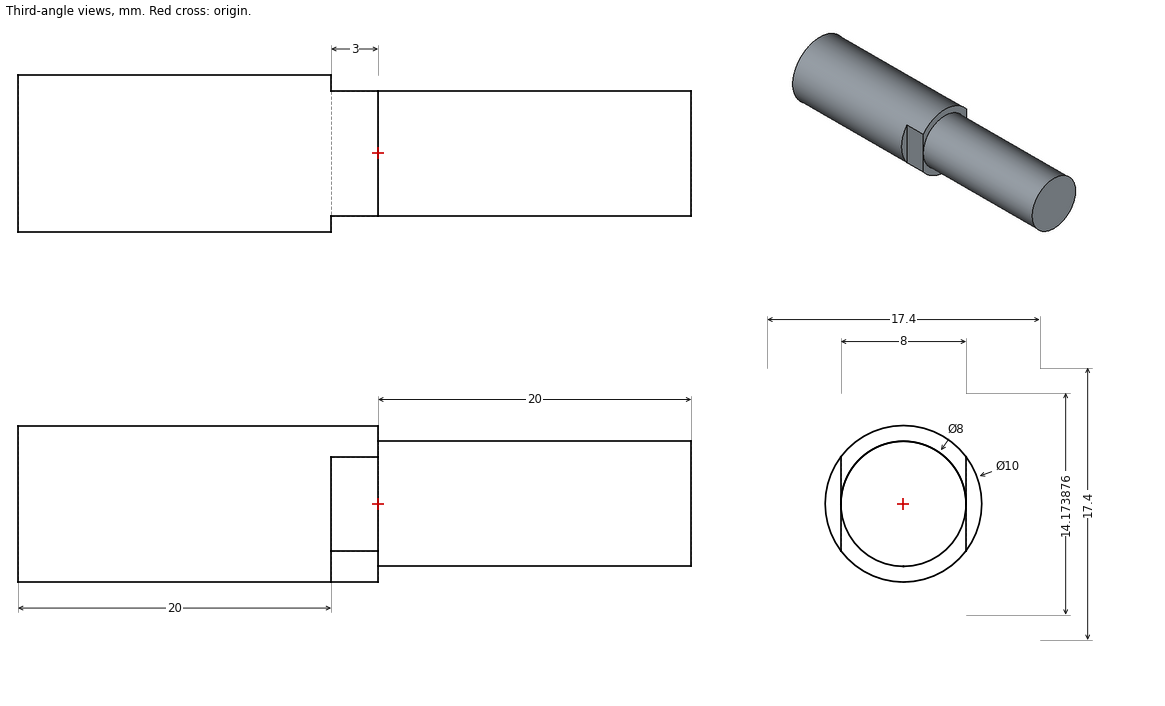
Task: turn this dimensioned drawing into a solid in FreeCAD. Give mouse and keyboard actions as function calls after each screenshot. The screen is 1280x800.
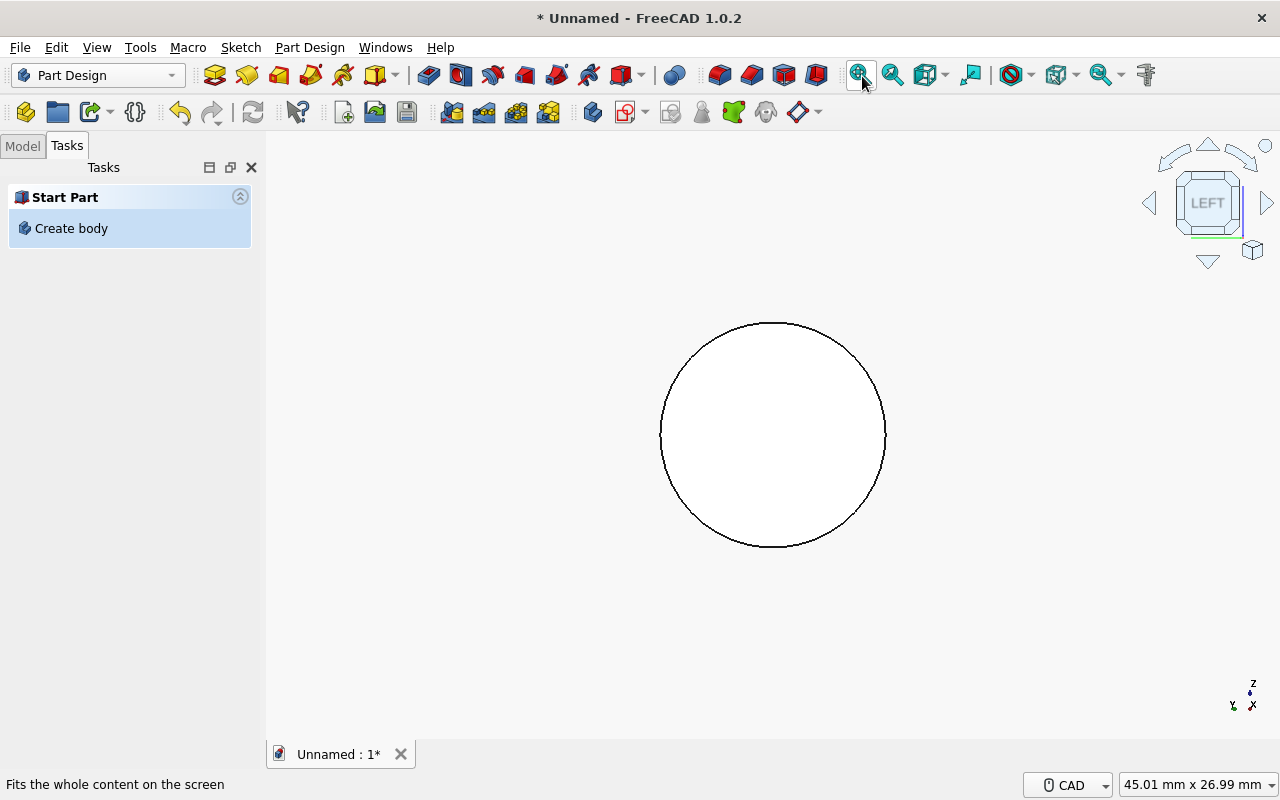
click(773, 434)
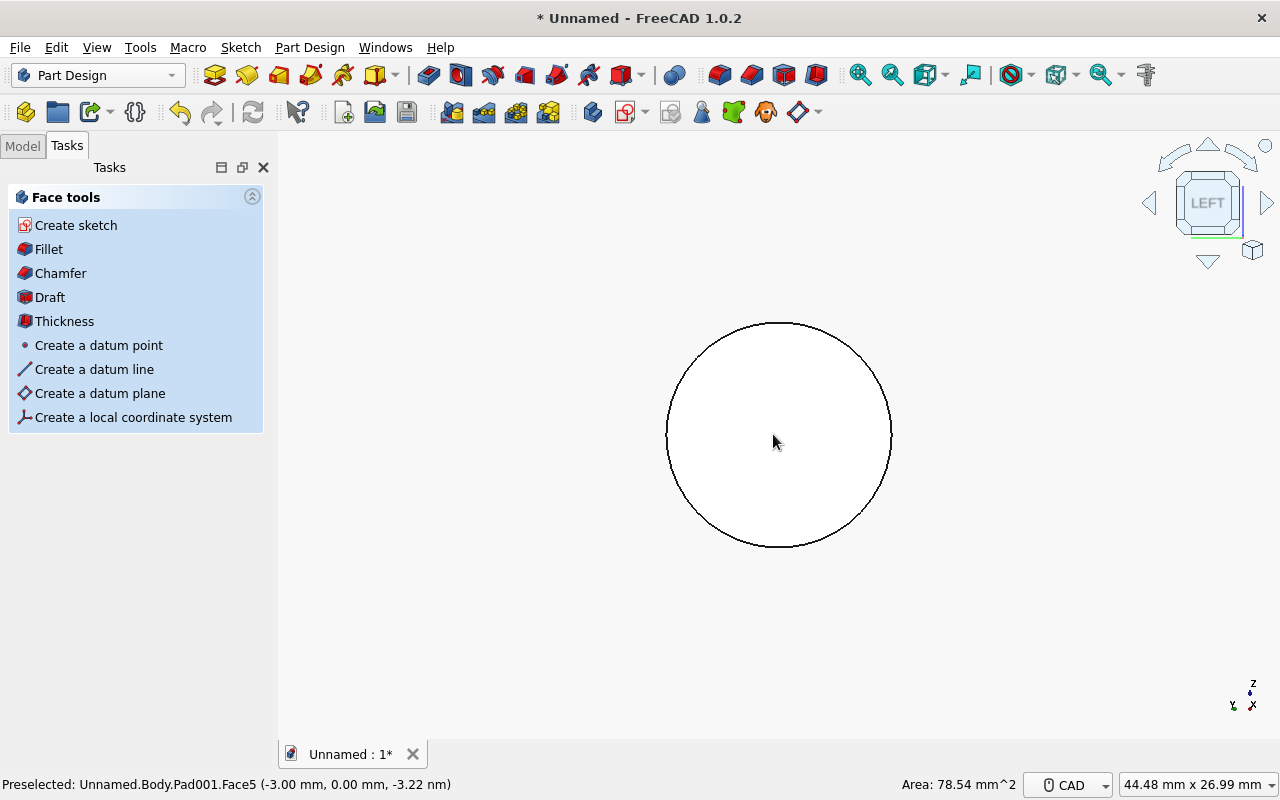
click(626, 112)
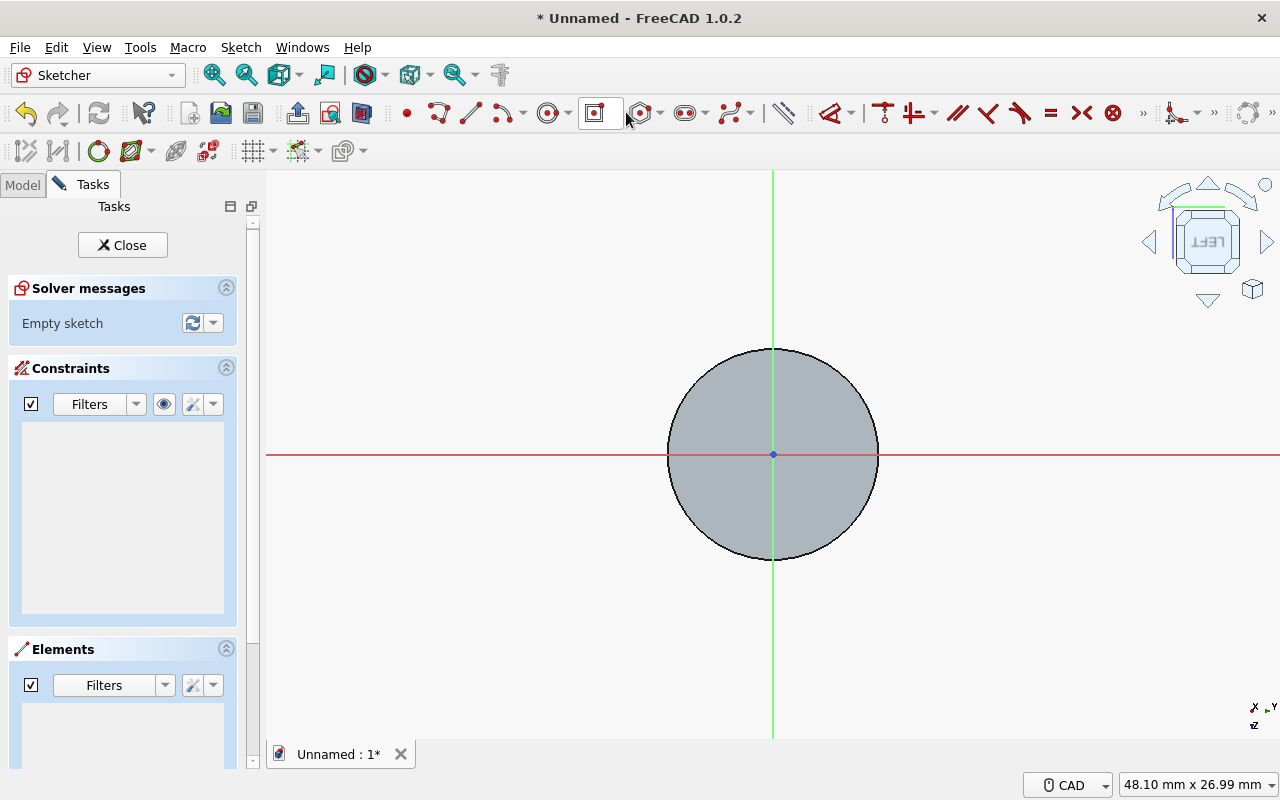
key(g)
key(v)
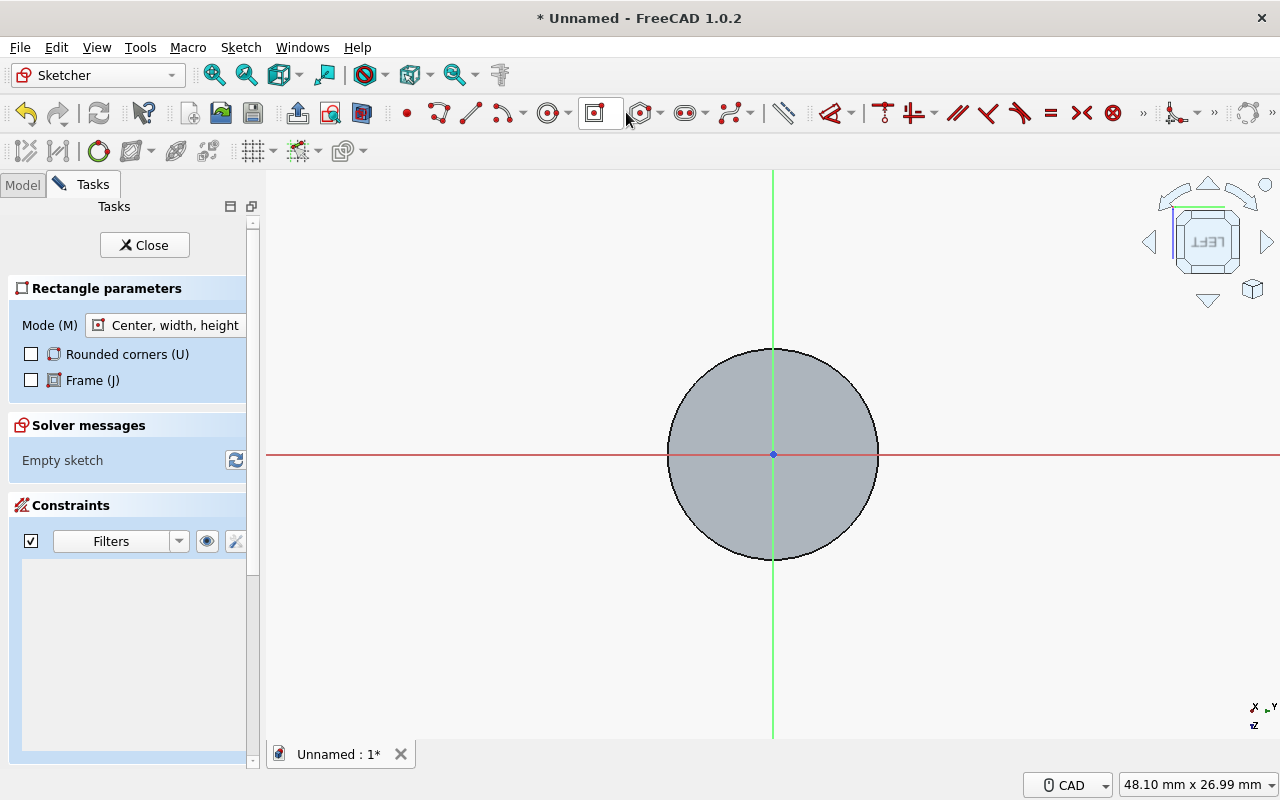
click(773, 454)
click(956, 271)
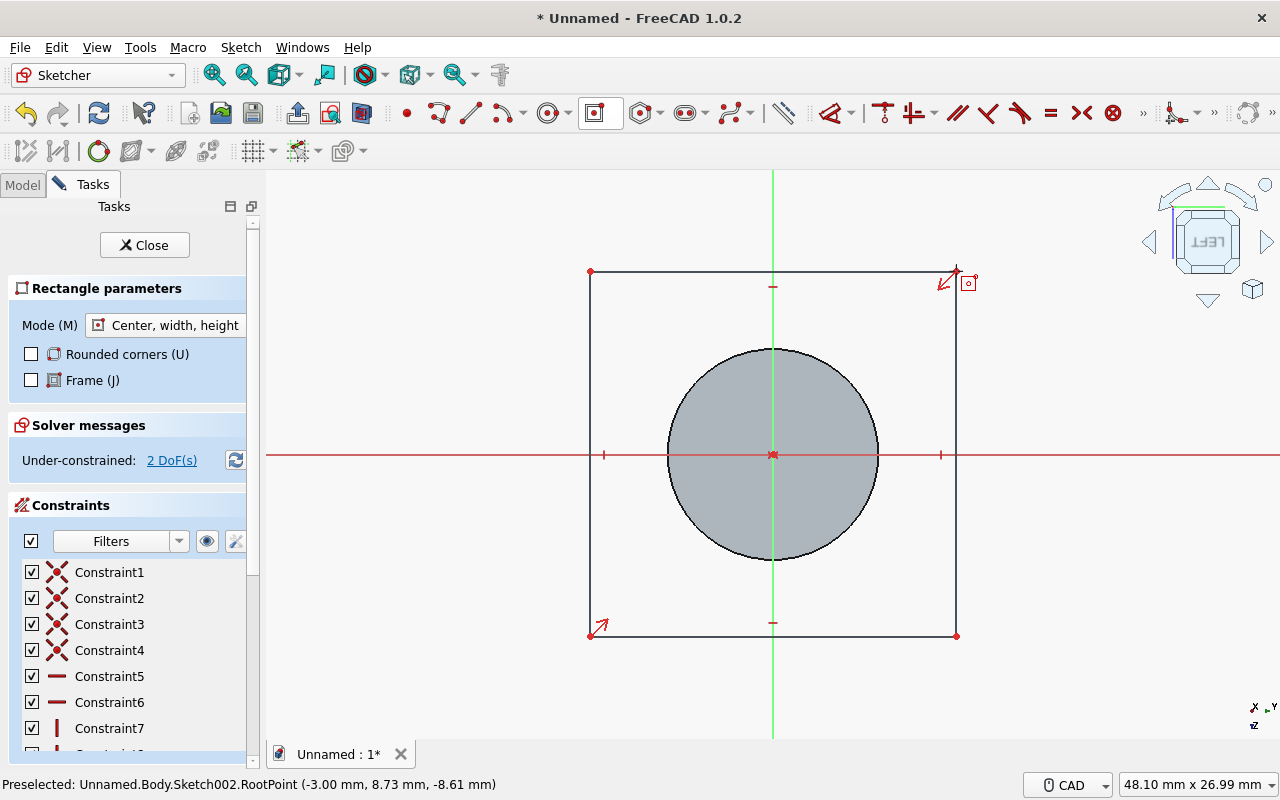
click(773, 454)
click(857, 305)
key(Escape)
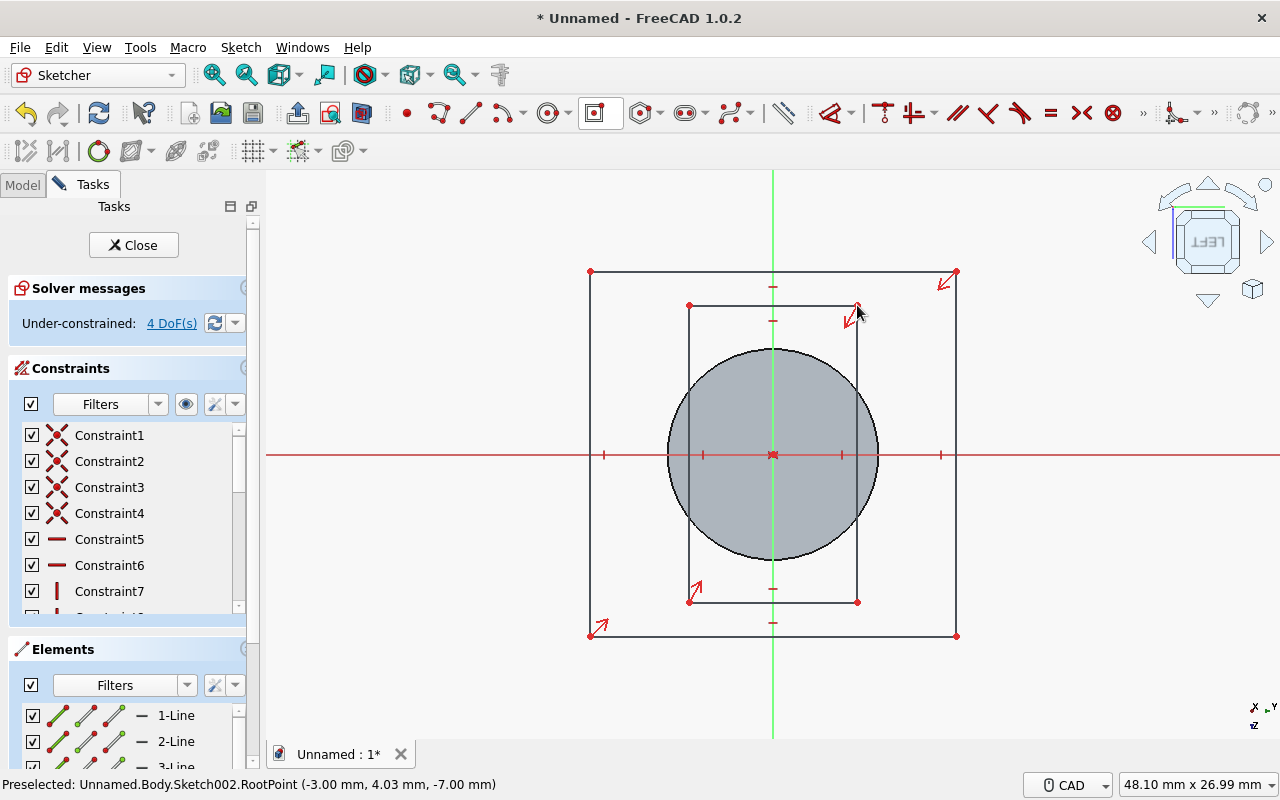
click(739, 603)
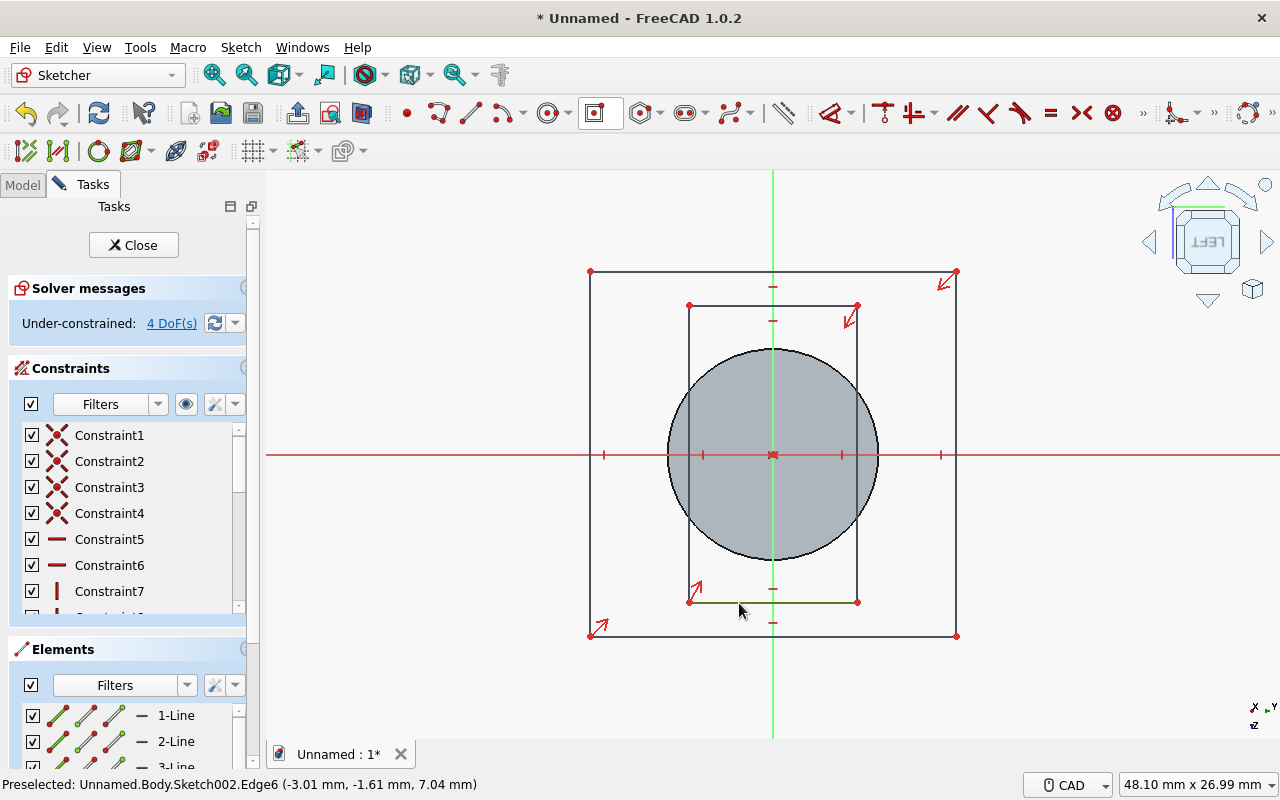
key(l)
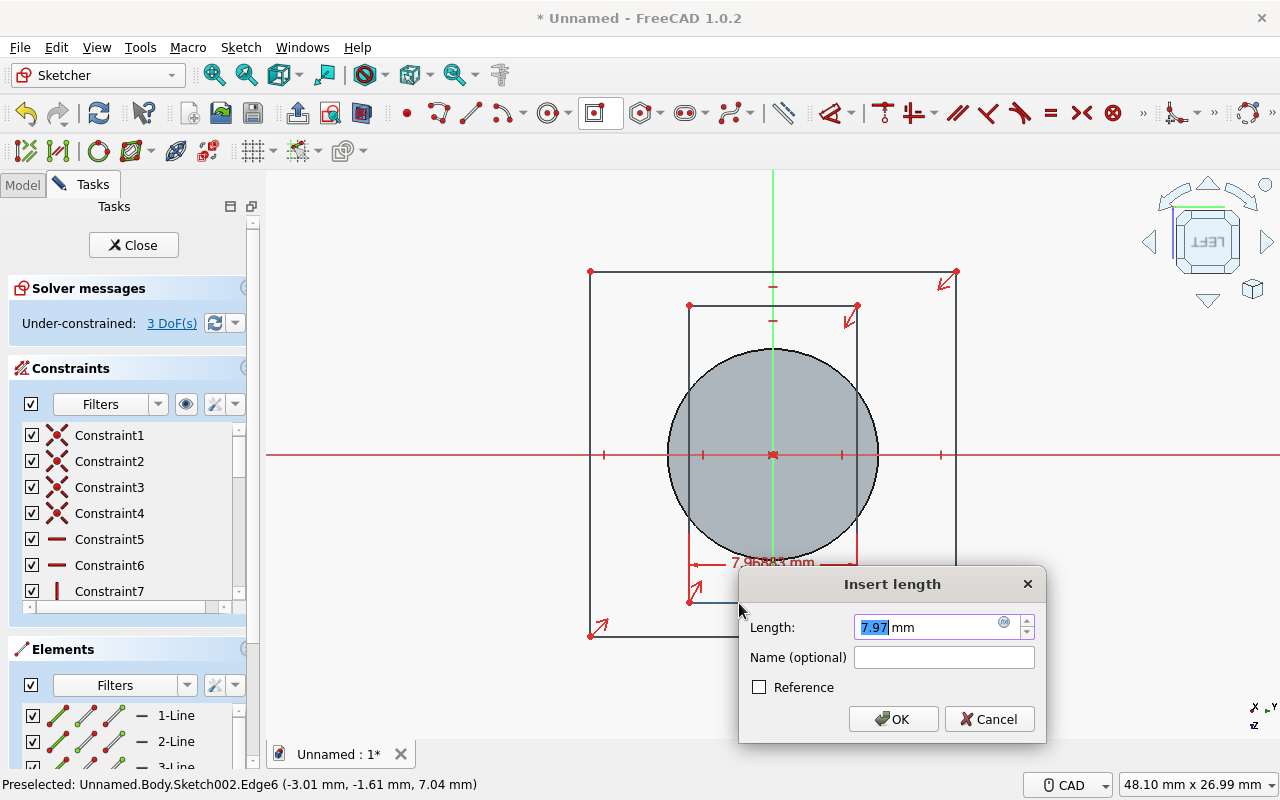
text(8)
key(Return)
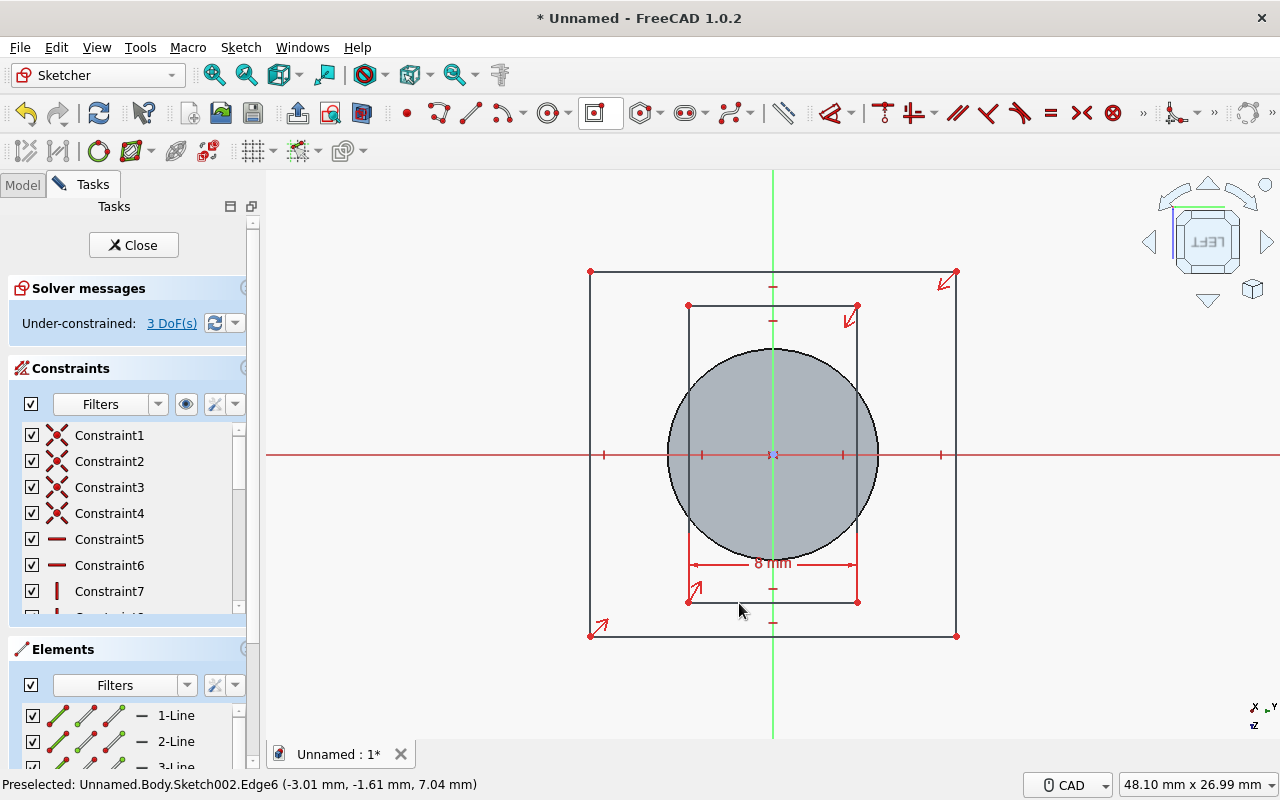
click(700, 637)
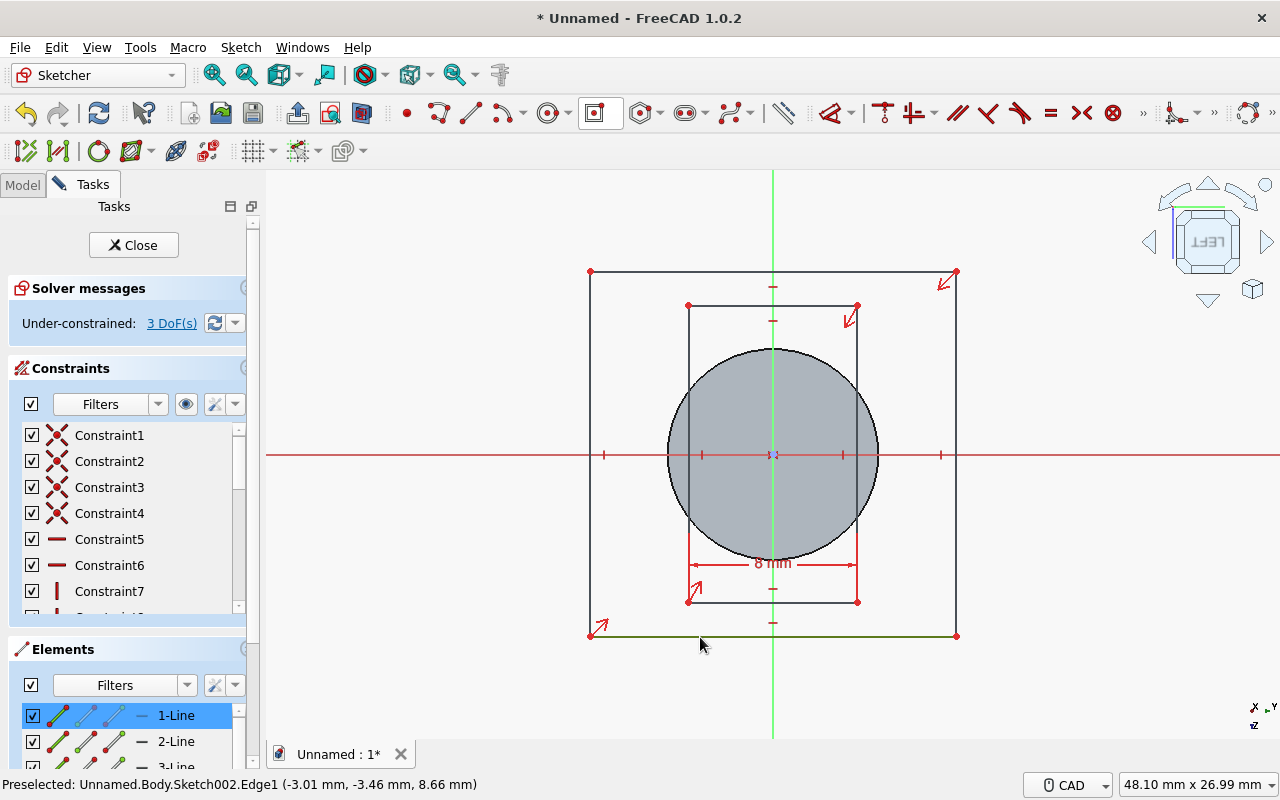
click(854, 114)